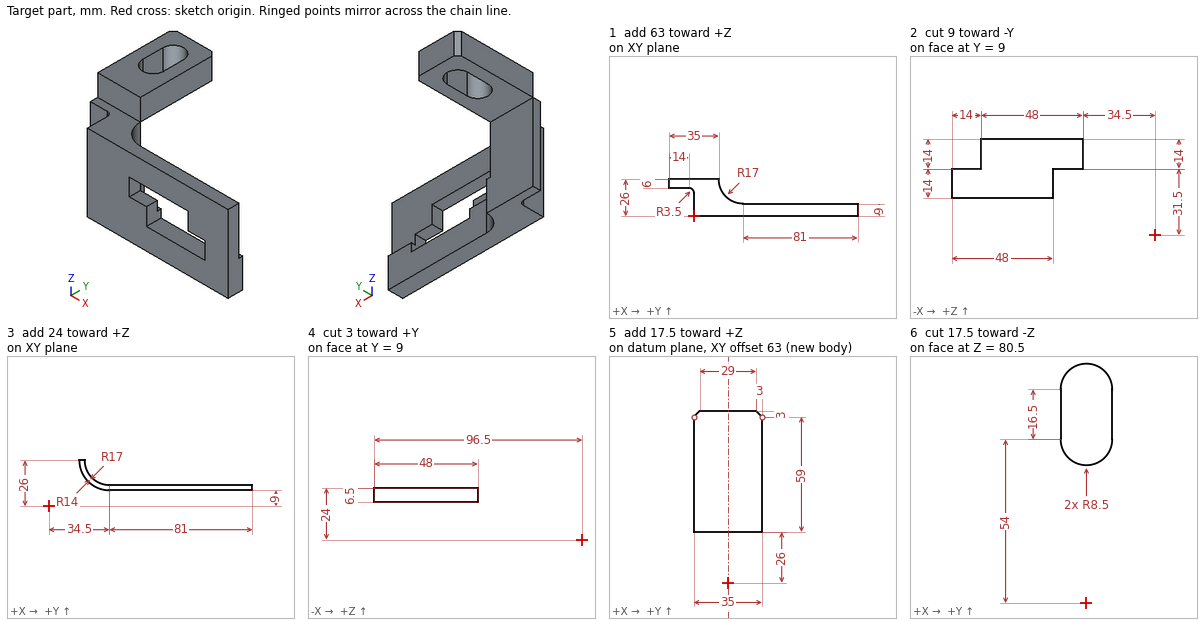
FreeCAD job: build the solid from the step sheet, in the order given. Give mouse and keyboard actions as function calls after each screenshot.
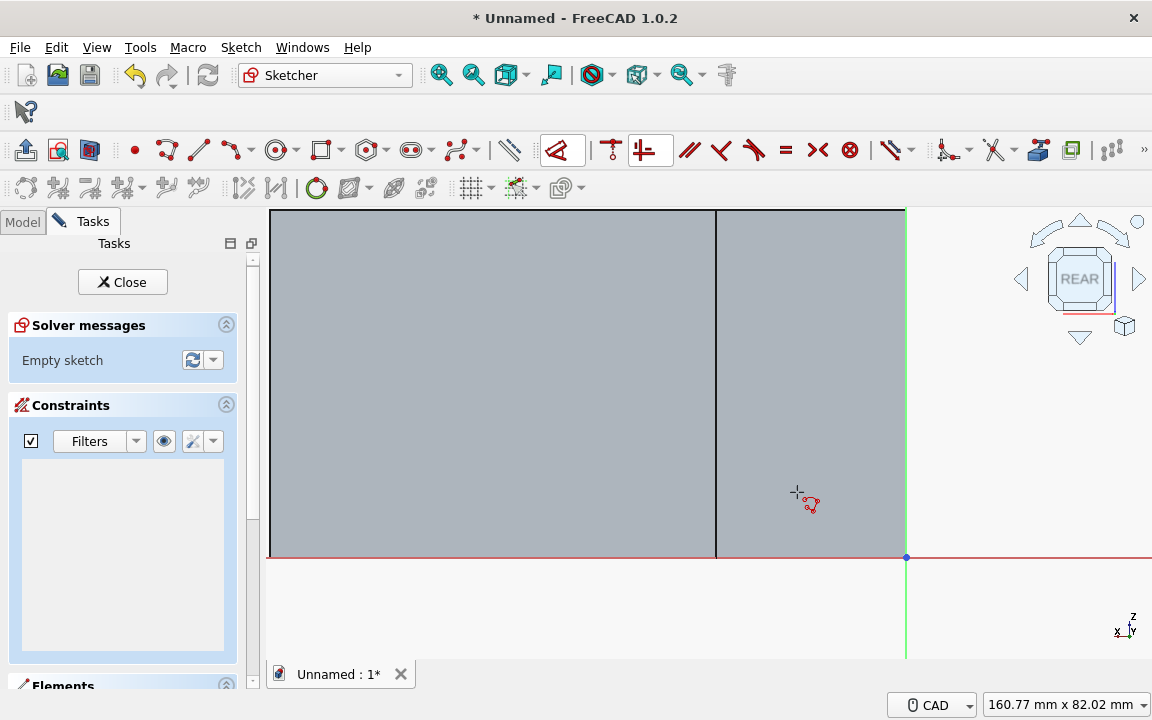
click(716, 384)
click(716, 307)
click(452, 307)
click(452, 384)
click(374, 384)
click(374, 461)
click(639, 461)
click(639, 384)
click(716, 385)
key(Escape)
key(Escape)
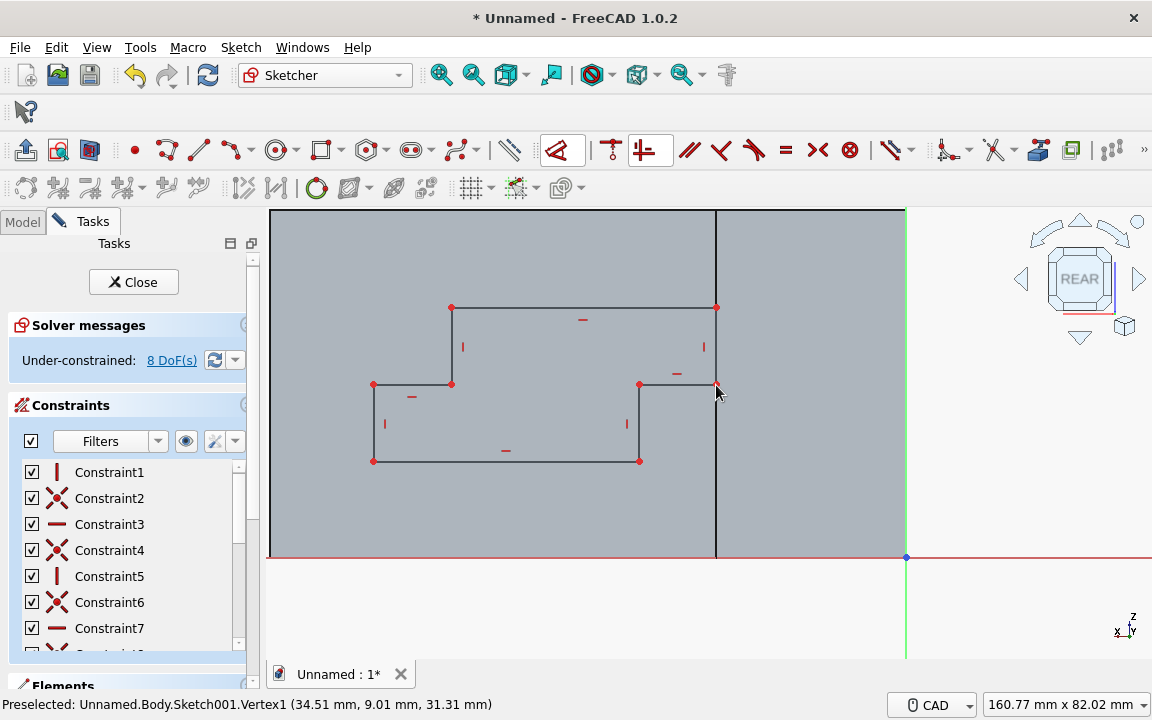
click(716, 362)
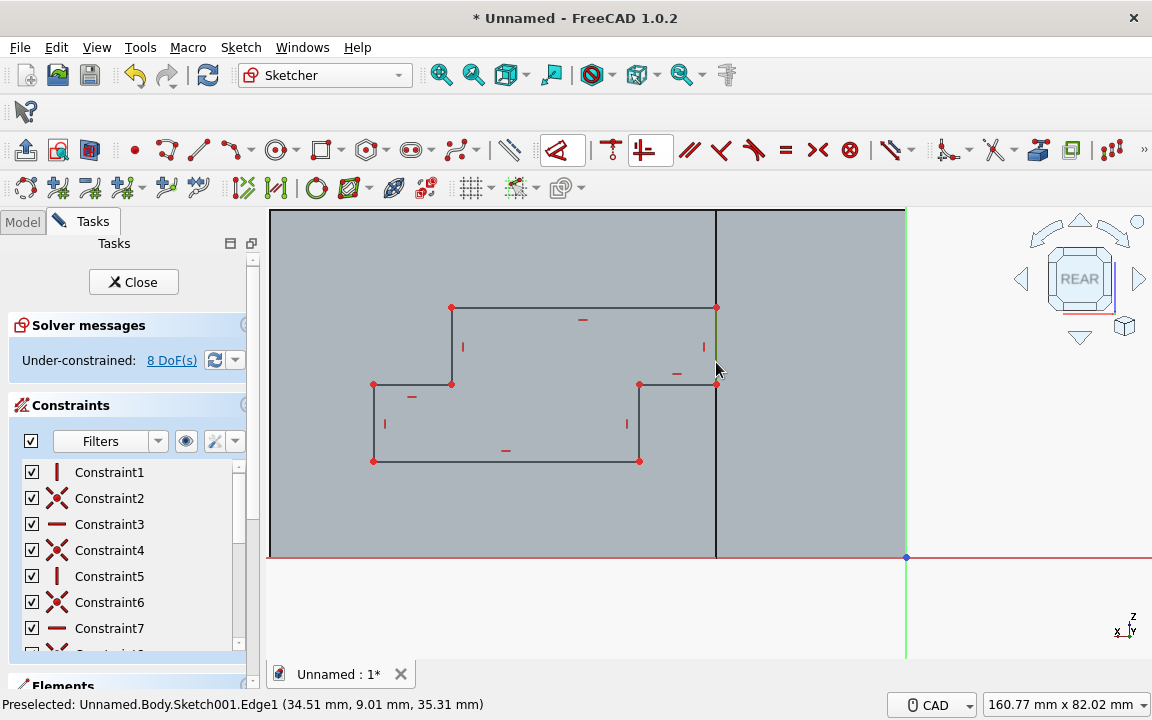
key(i)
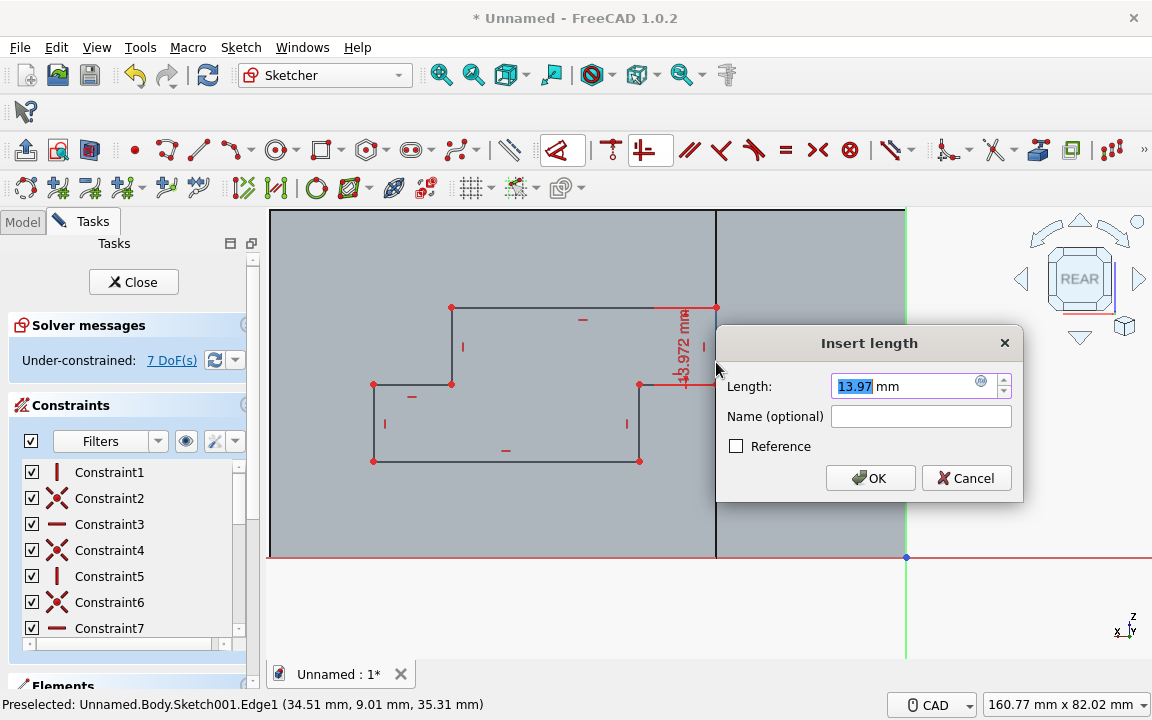
text(14)
key(Return)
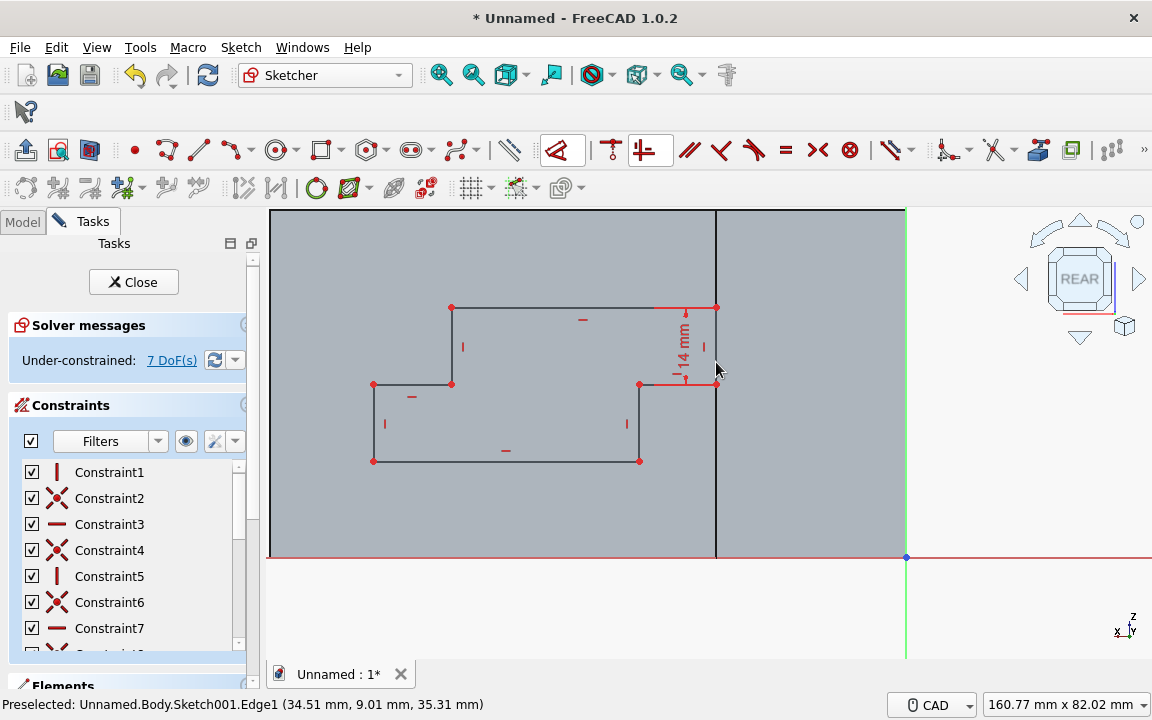
click(637, 308)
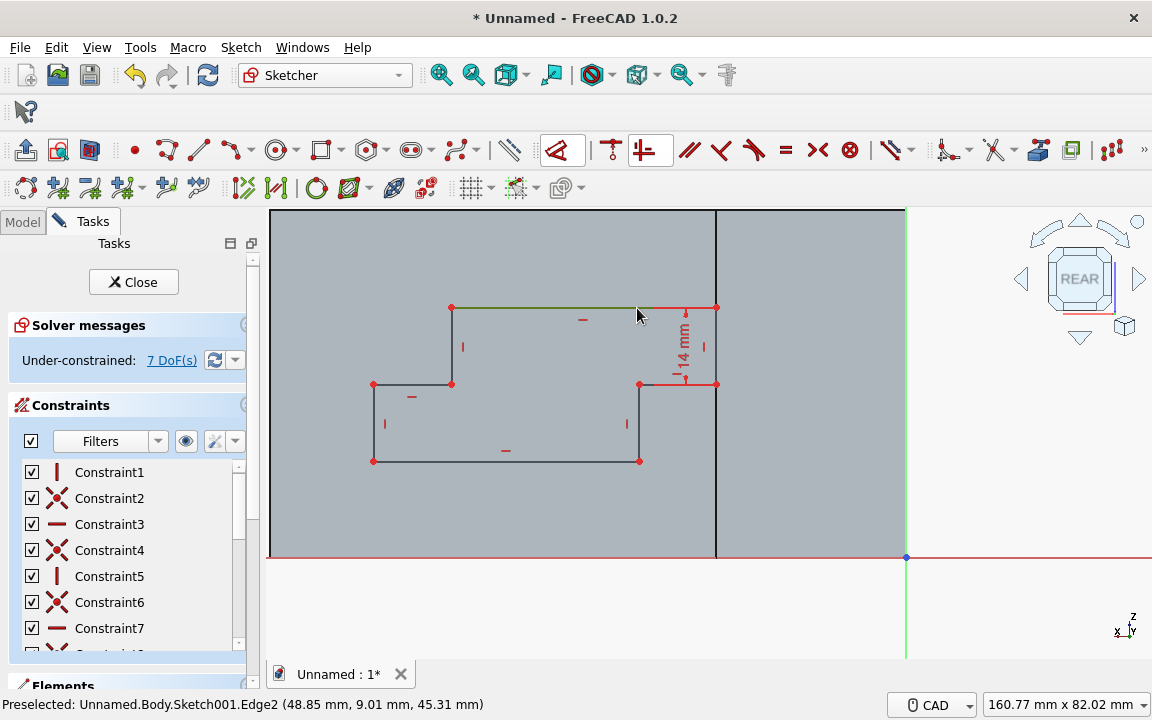
key(l)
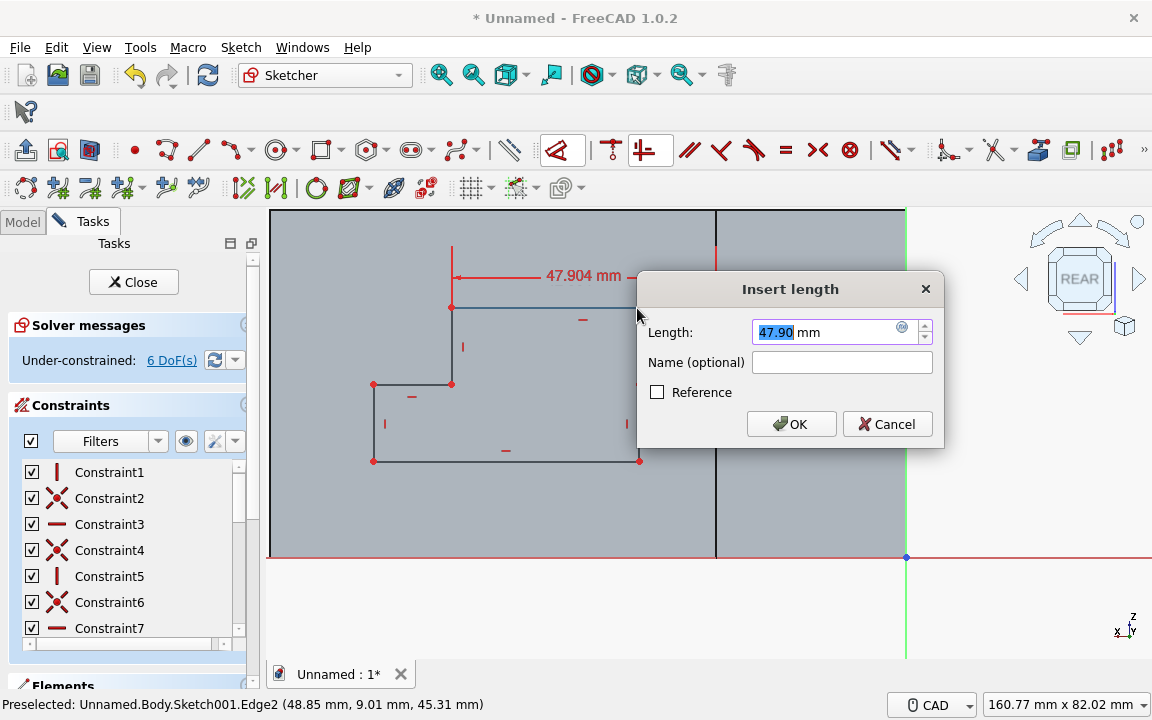
text(48)
key(Return)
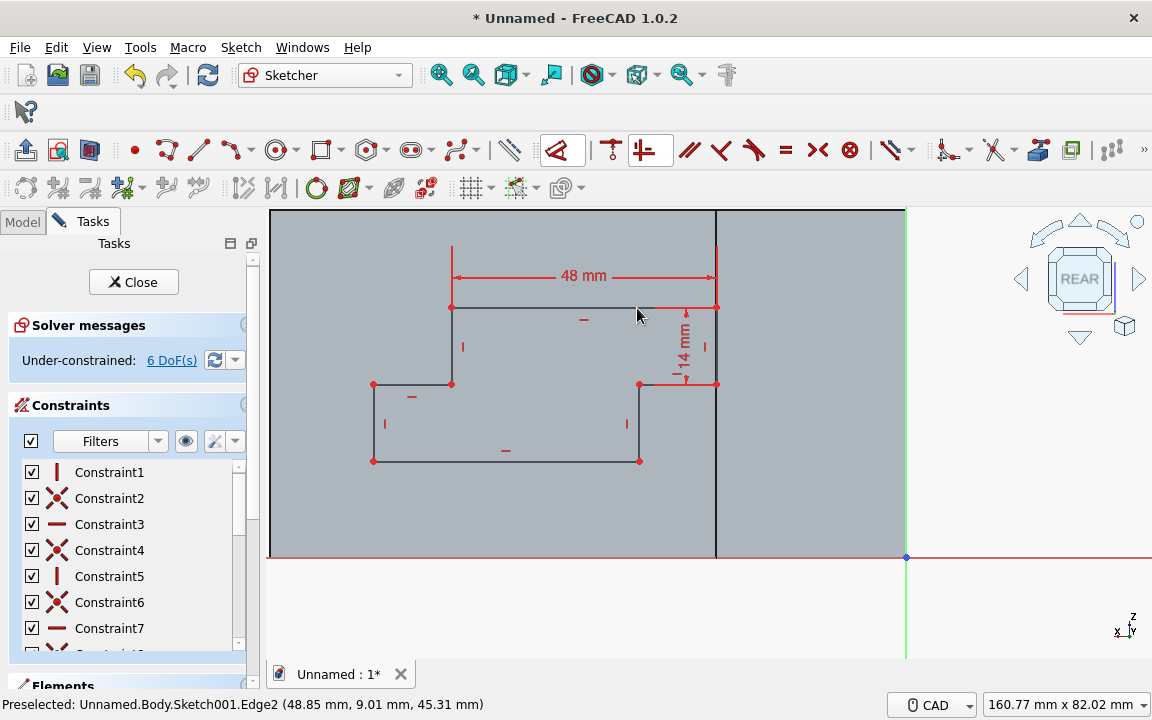
click(452, 331)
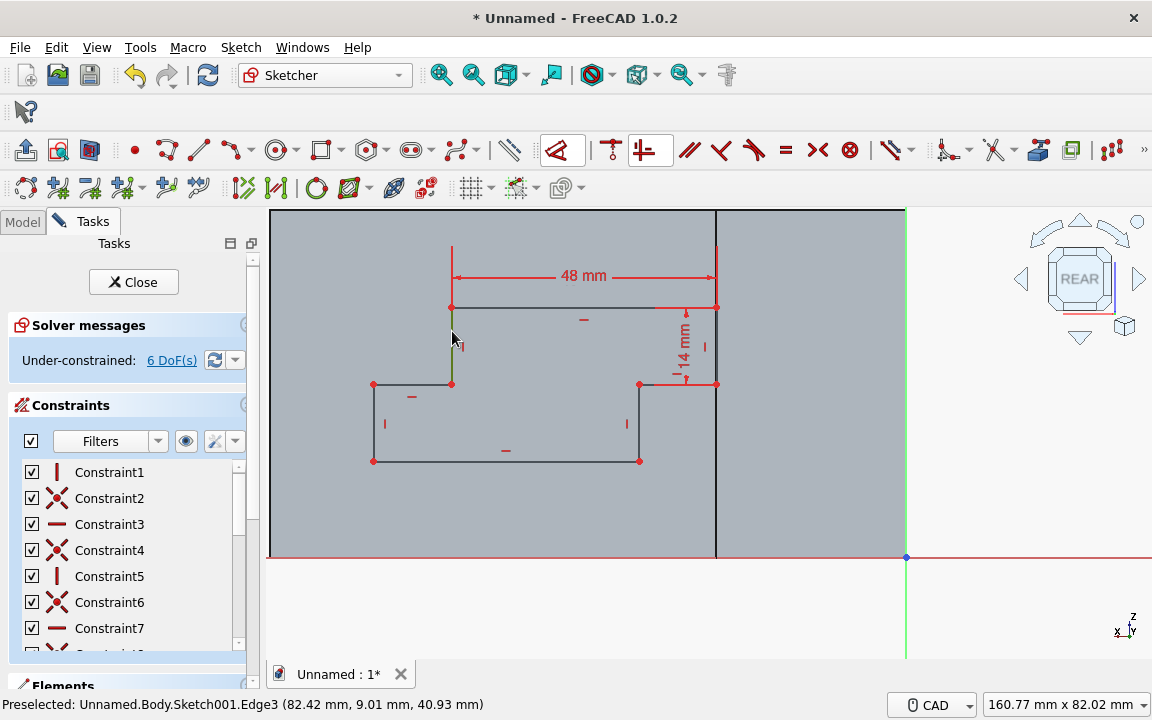
key(i)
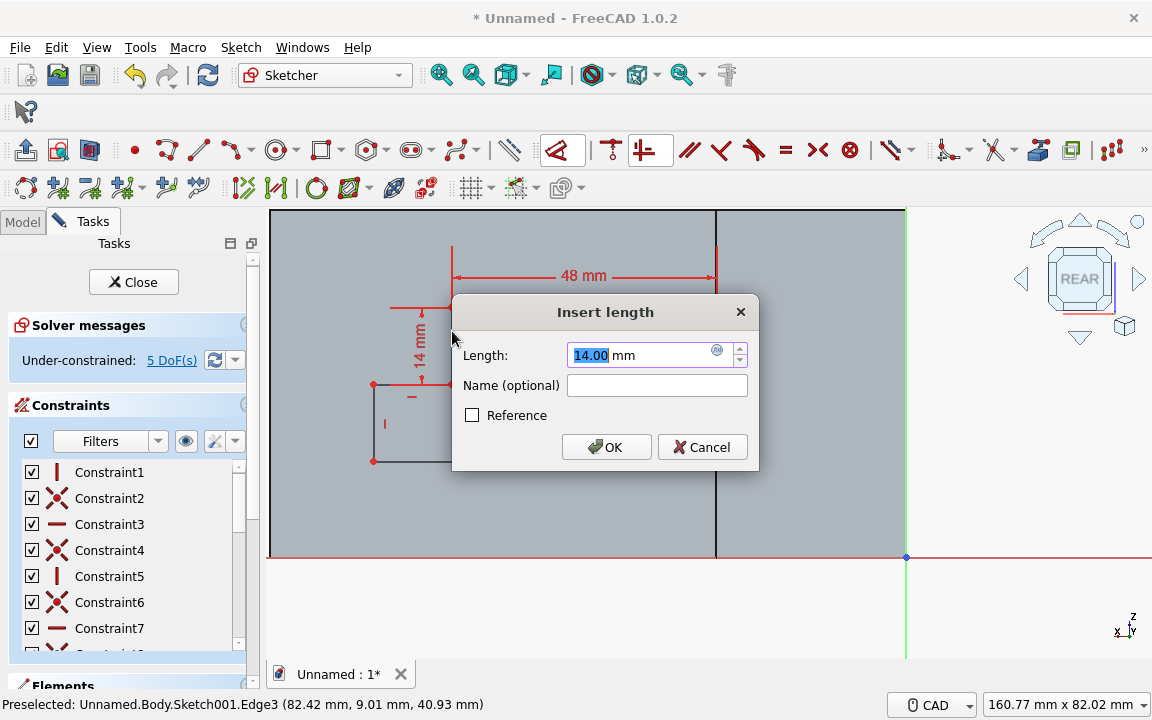
text(14)
key(Return)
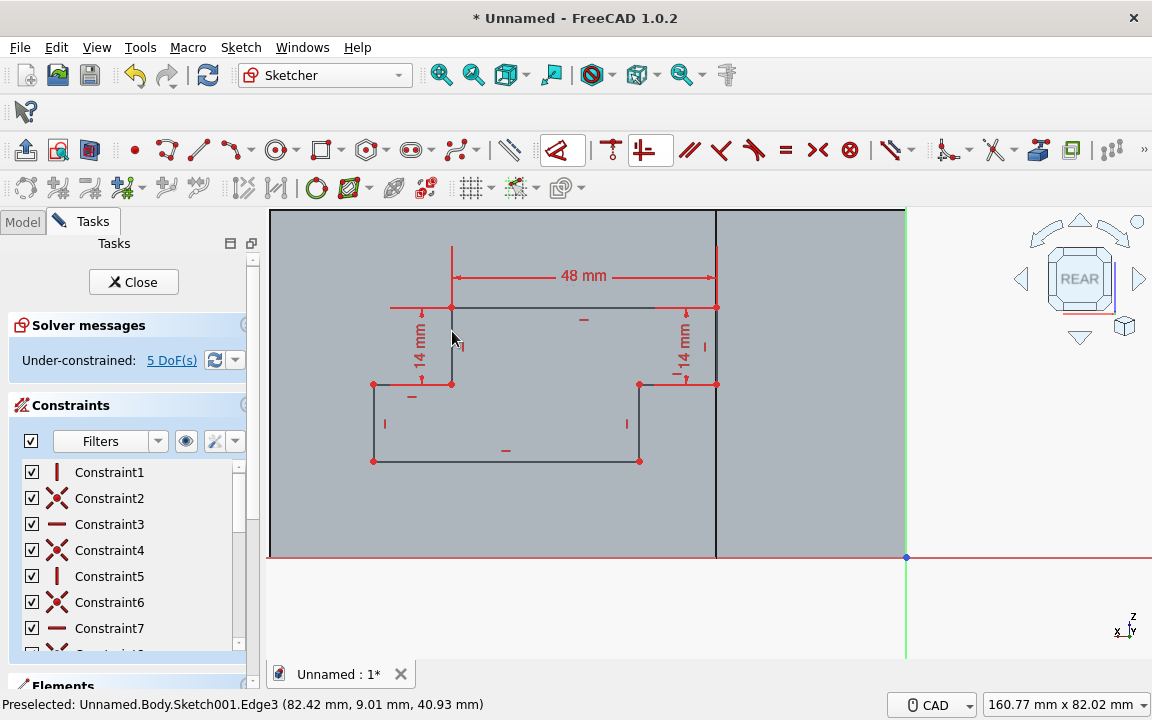
click(429, 385)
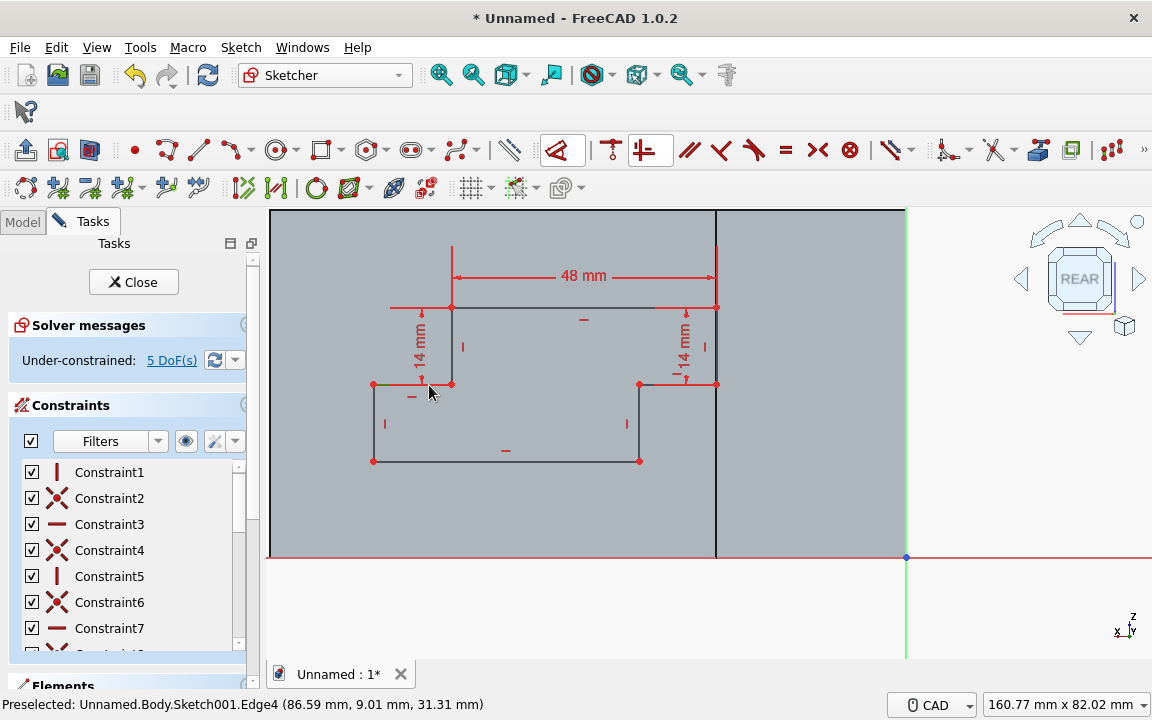
key(l)